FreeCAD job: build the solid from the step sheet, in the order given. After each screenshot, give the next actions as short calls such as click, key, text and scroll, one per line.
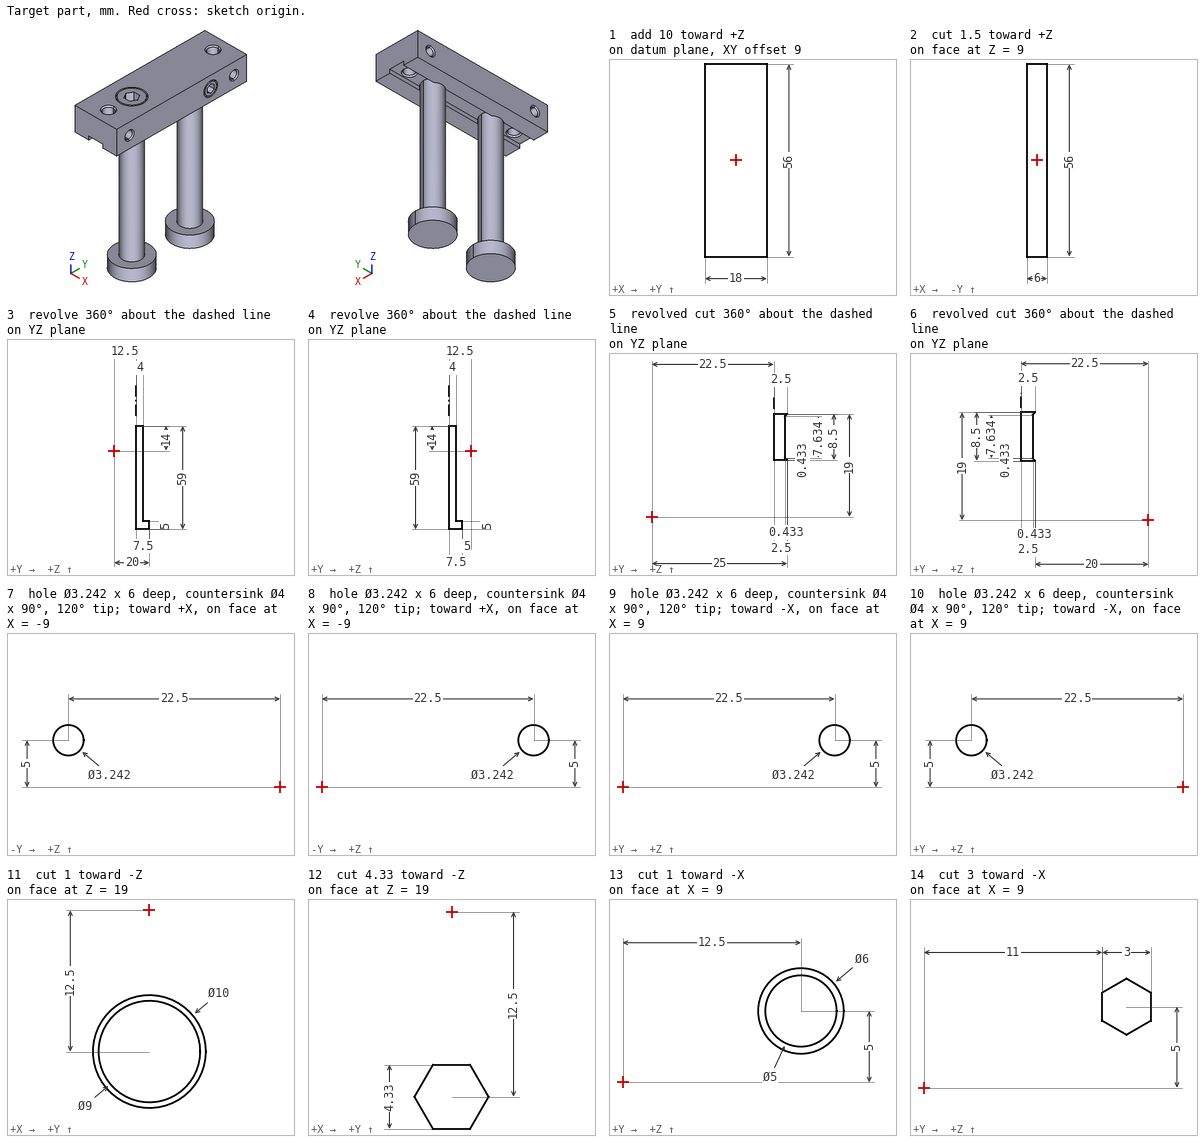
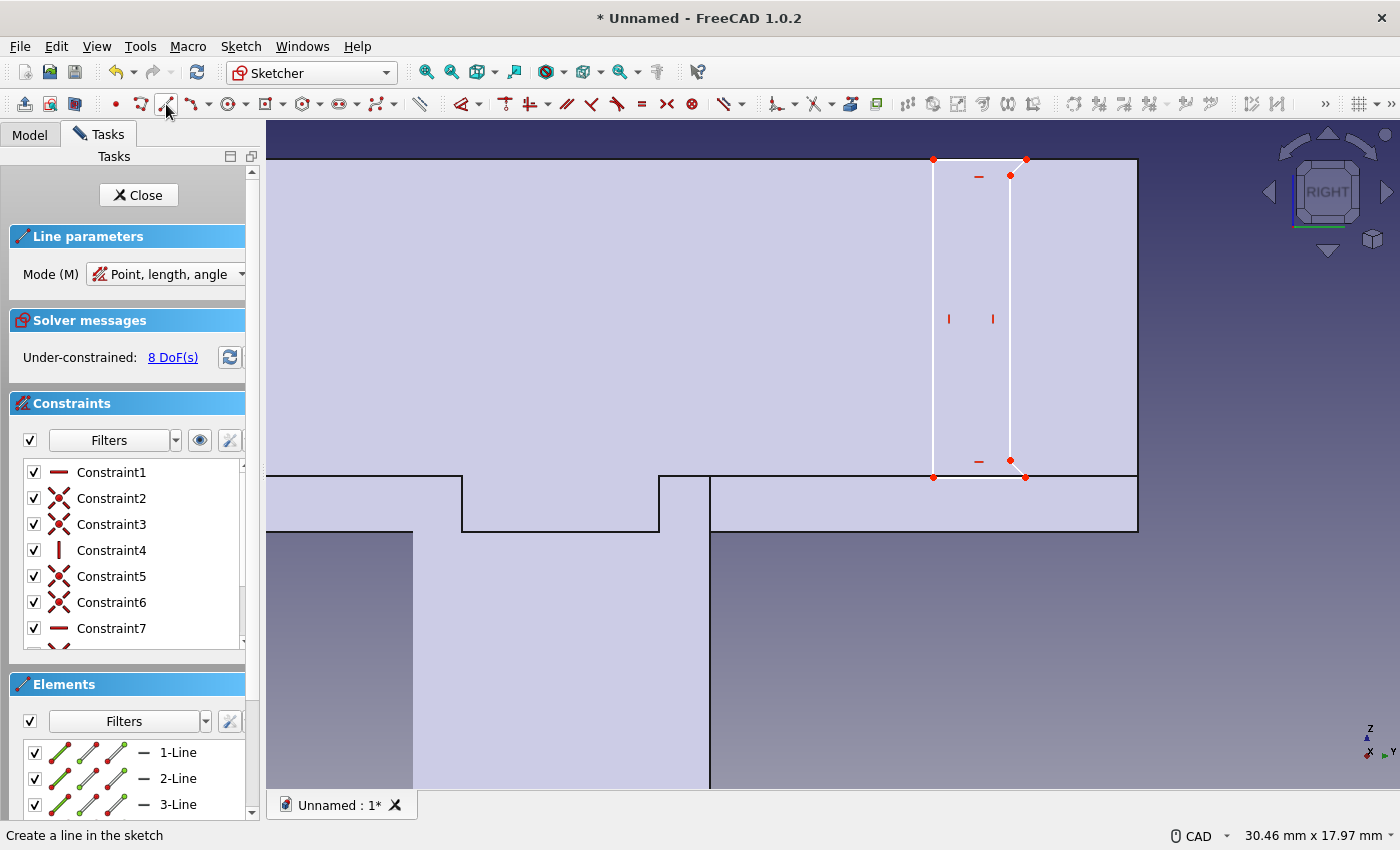
scroll(1012, 460, down, 3)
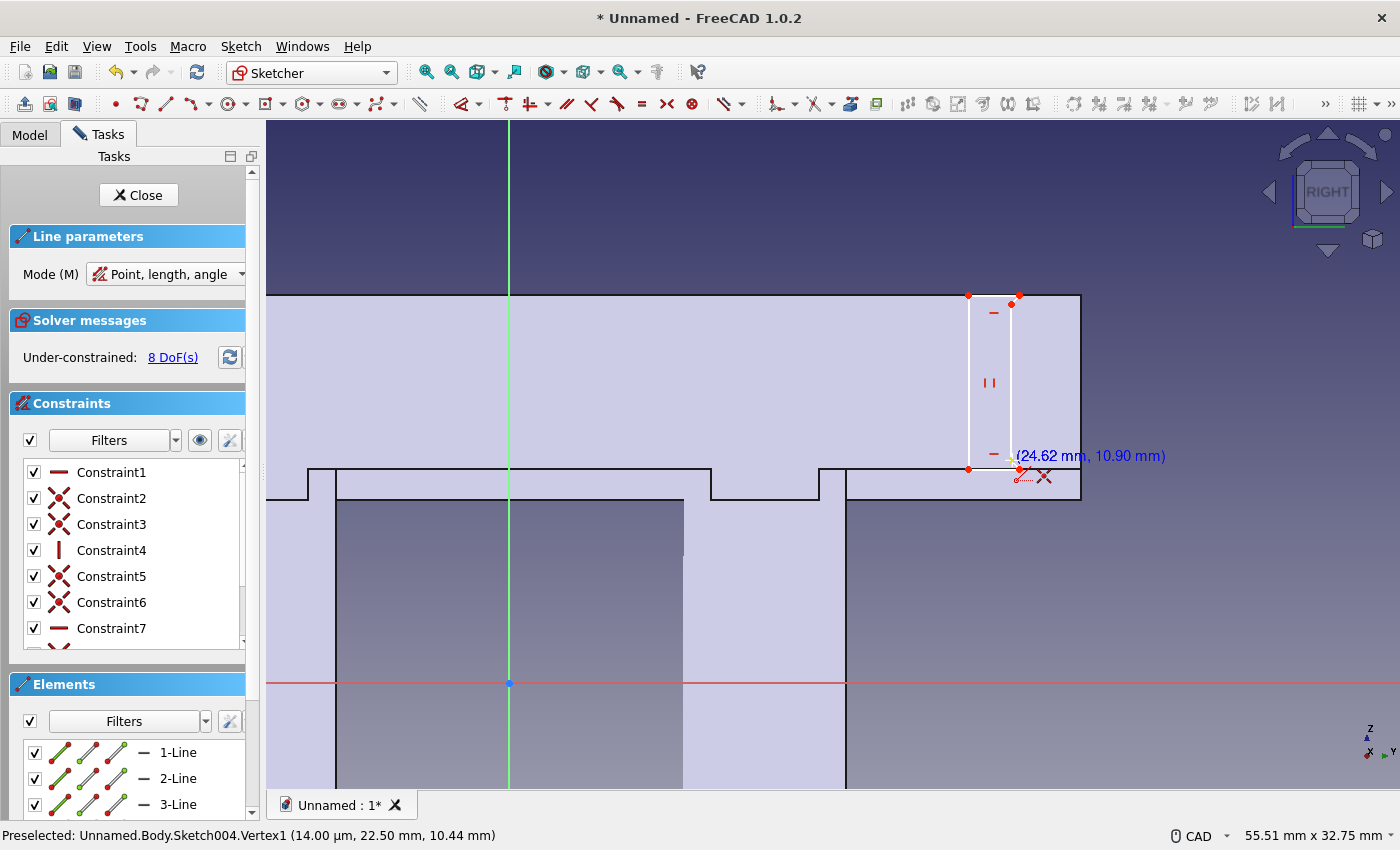
click(969, 278)
click(969, 226)
key(Escape)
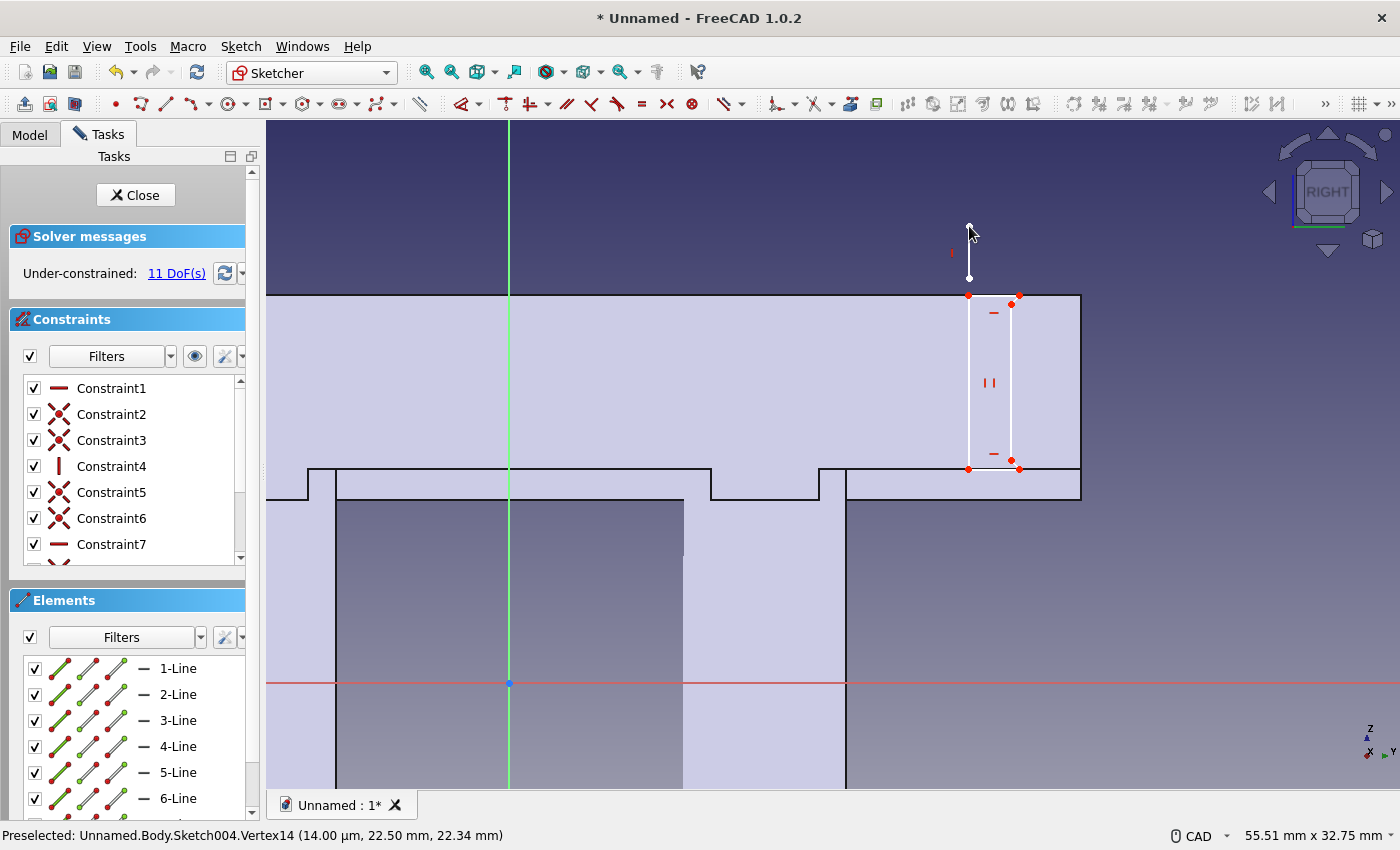
click(969, 263)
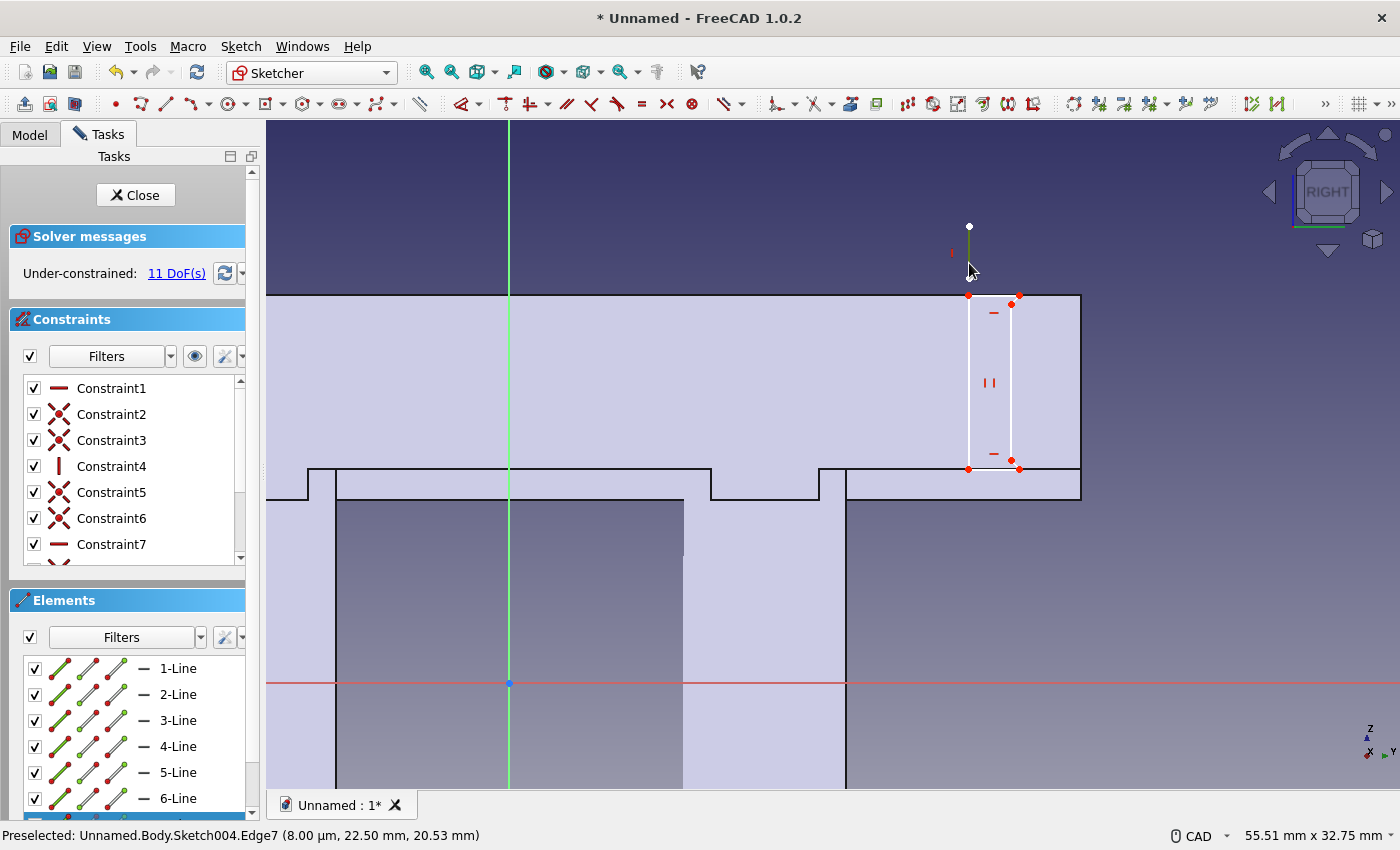
click(420, 104)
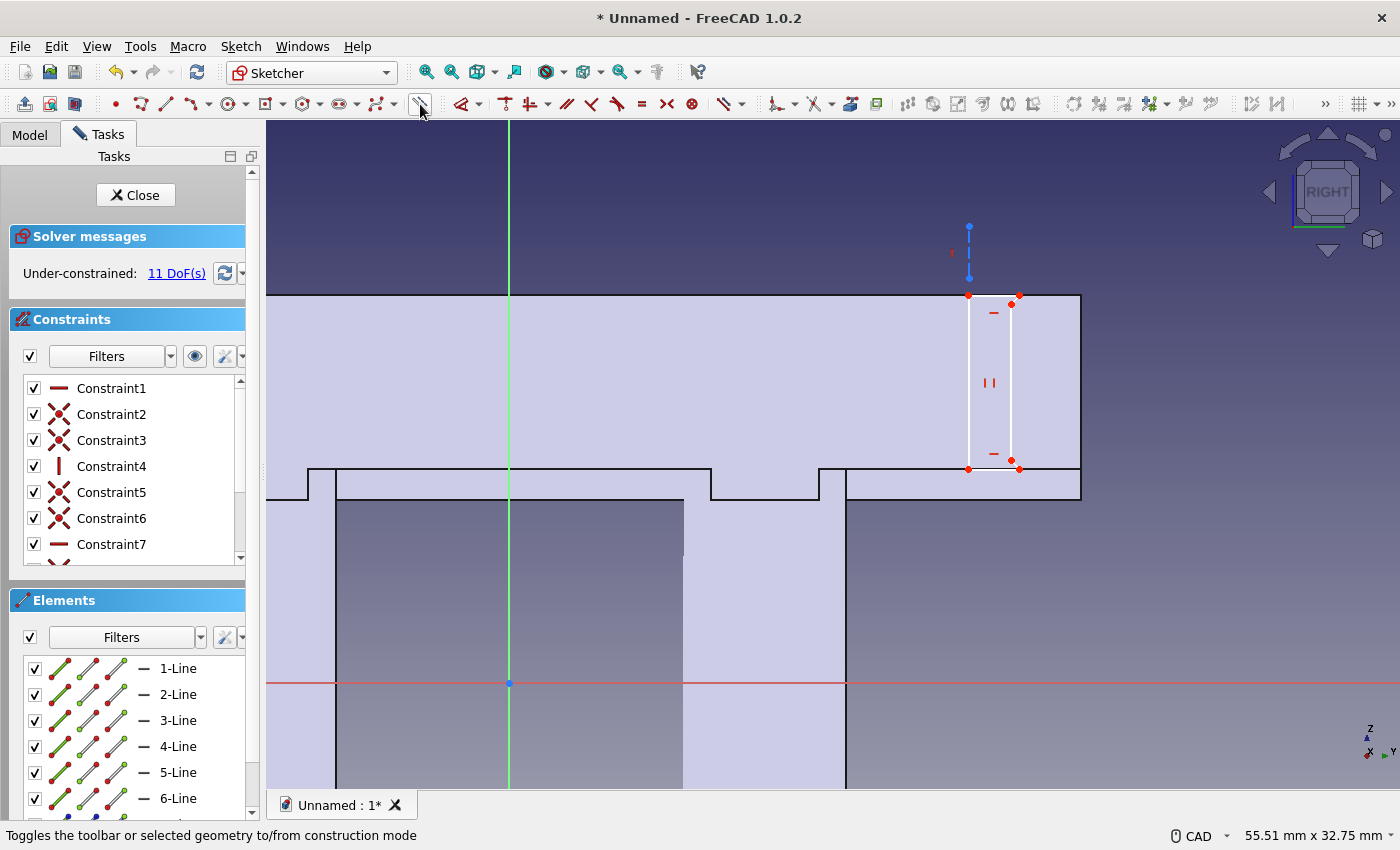
click(460, 104)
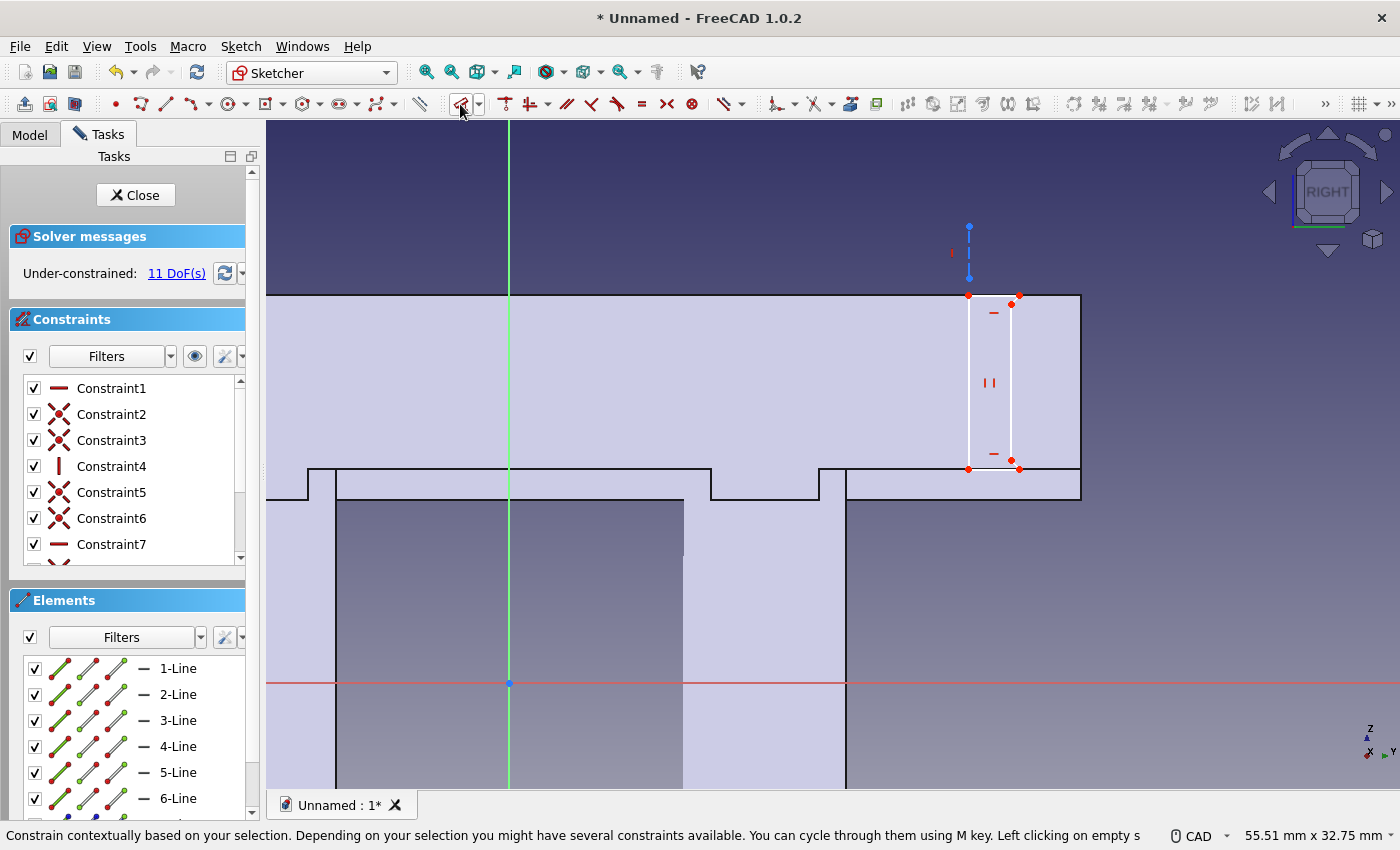
click(984, 470)
click(994, 504)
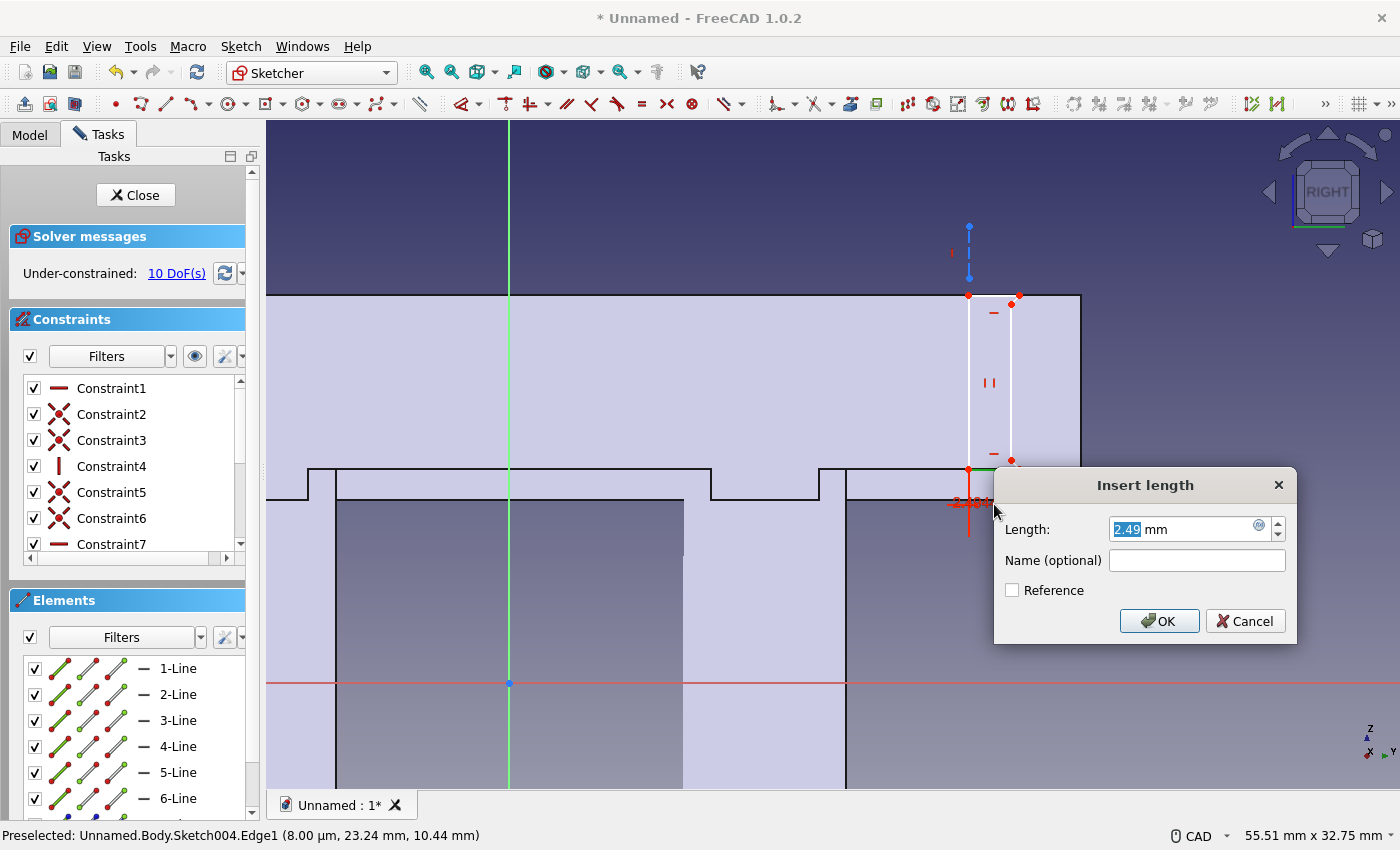
text(2.5)
key(Return)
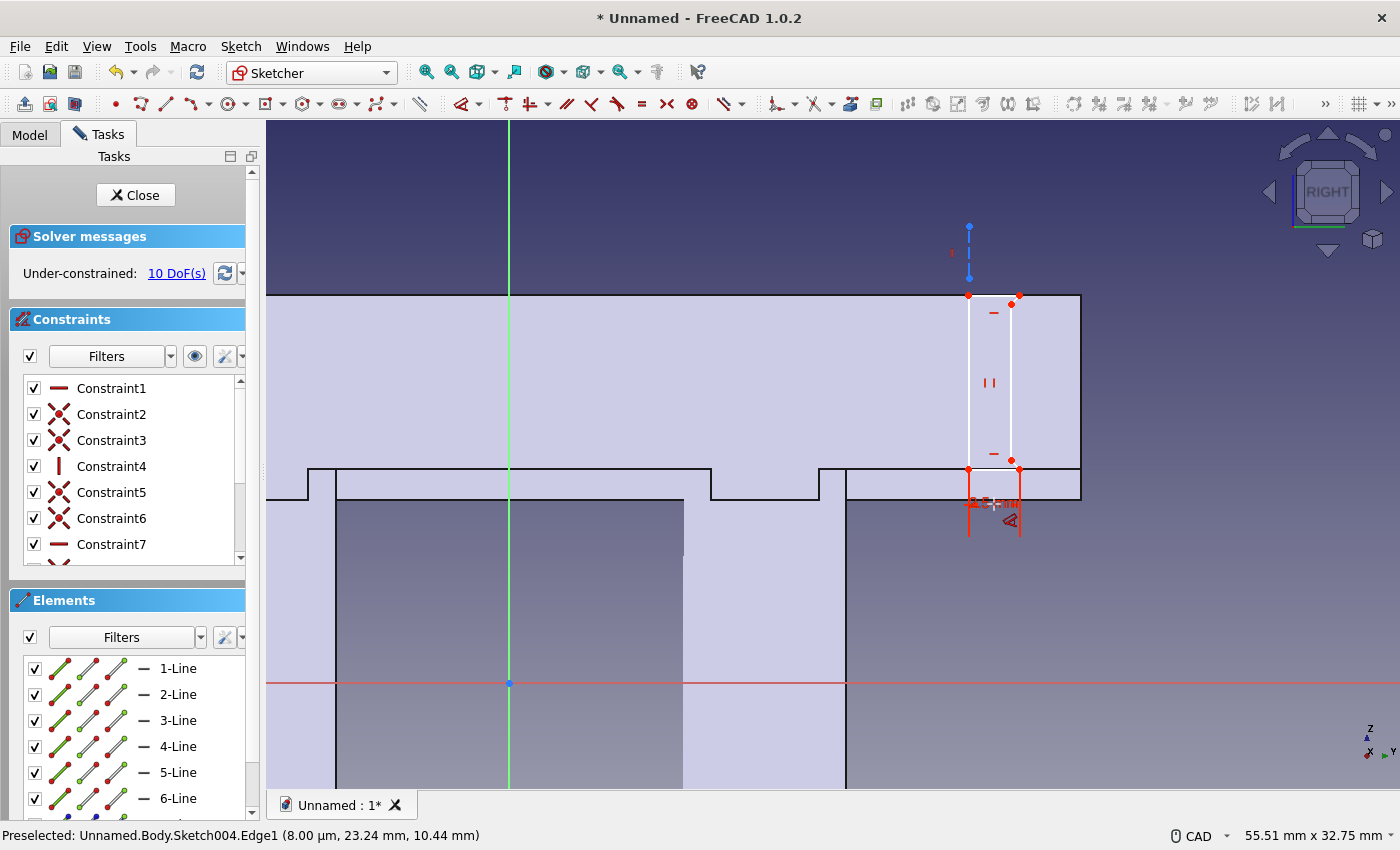
scroll(1005, 296, up, 2)